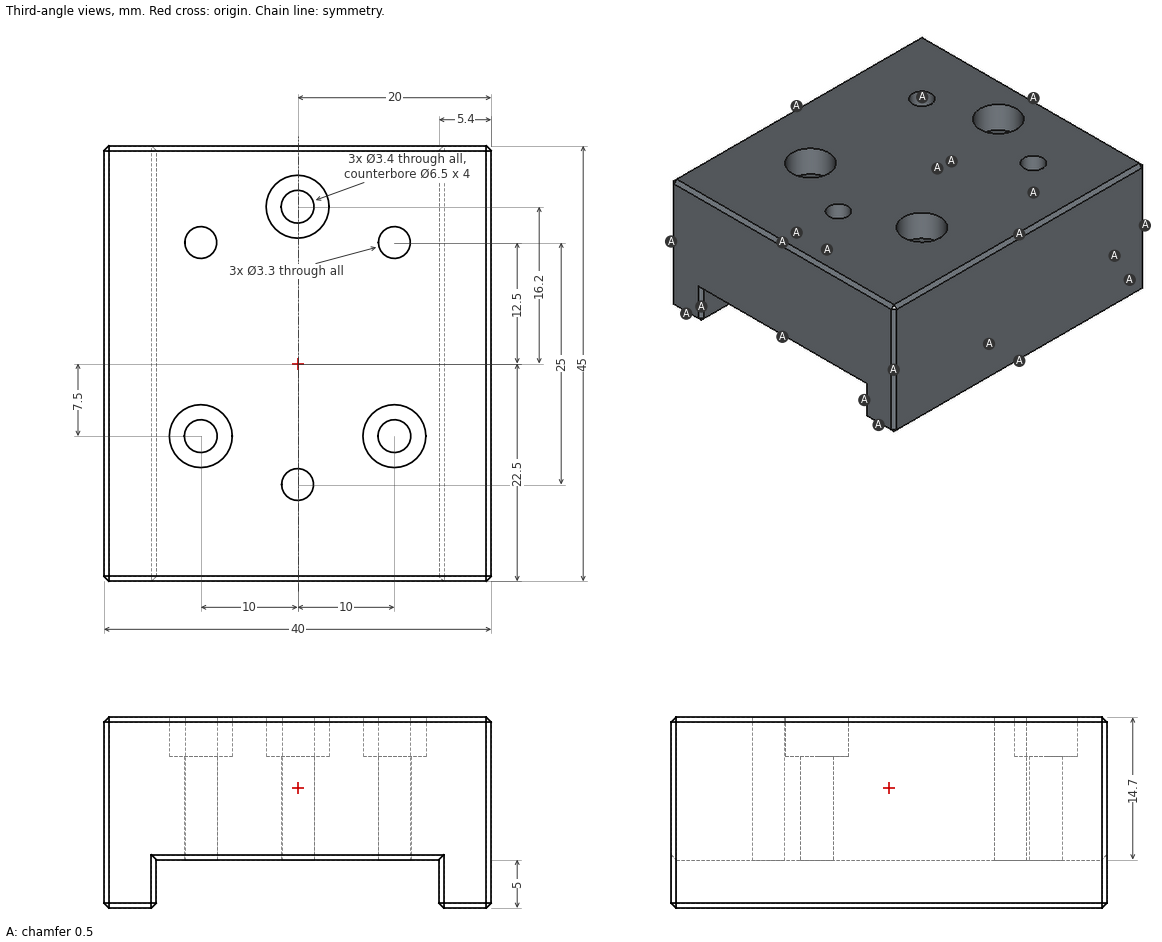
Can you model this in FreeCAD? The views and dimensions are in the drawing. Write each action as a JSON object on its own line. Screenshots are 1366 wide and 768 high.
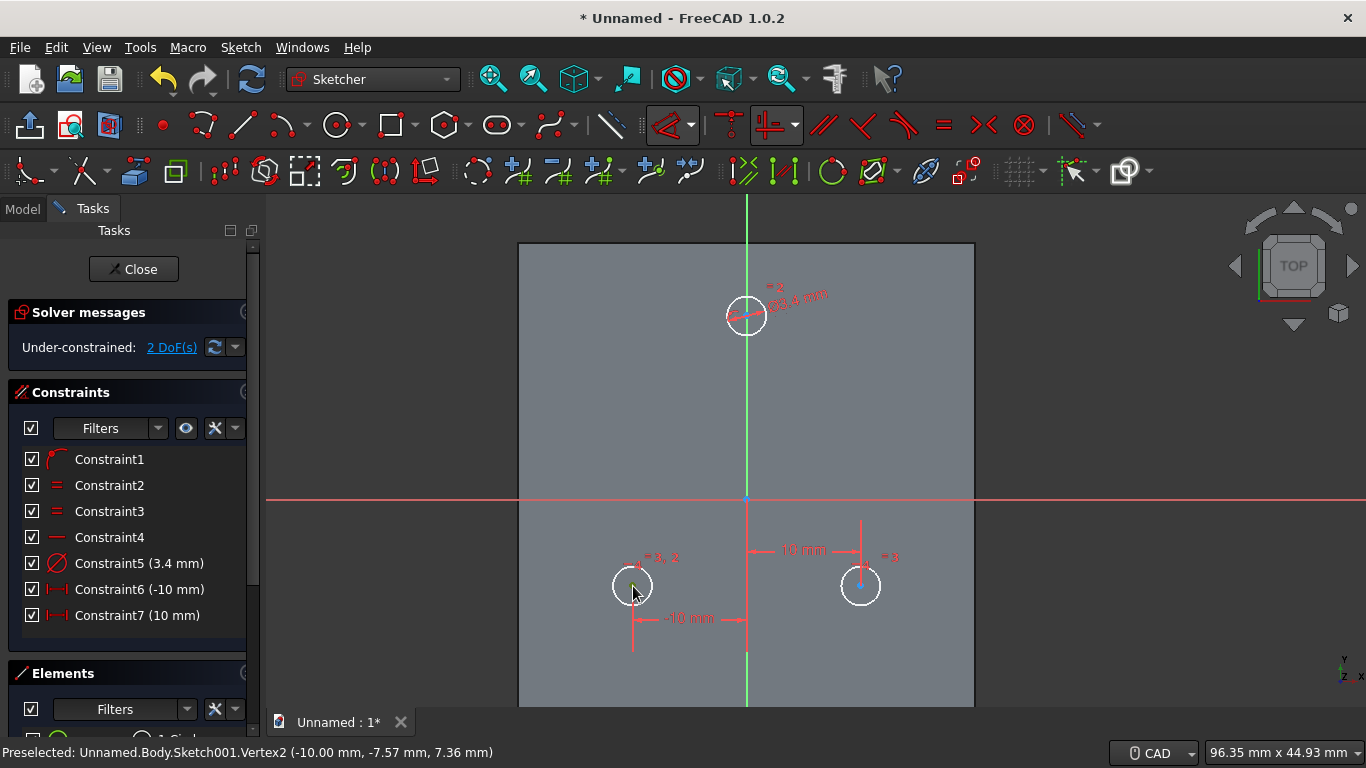
{"action": "key", "text": "i"}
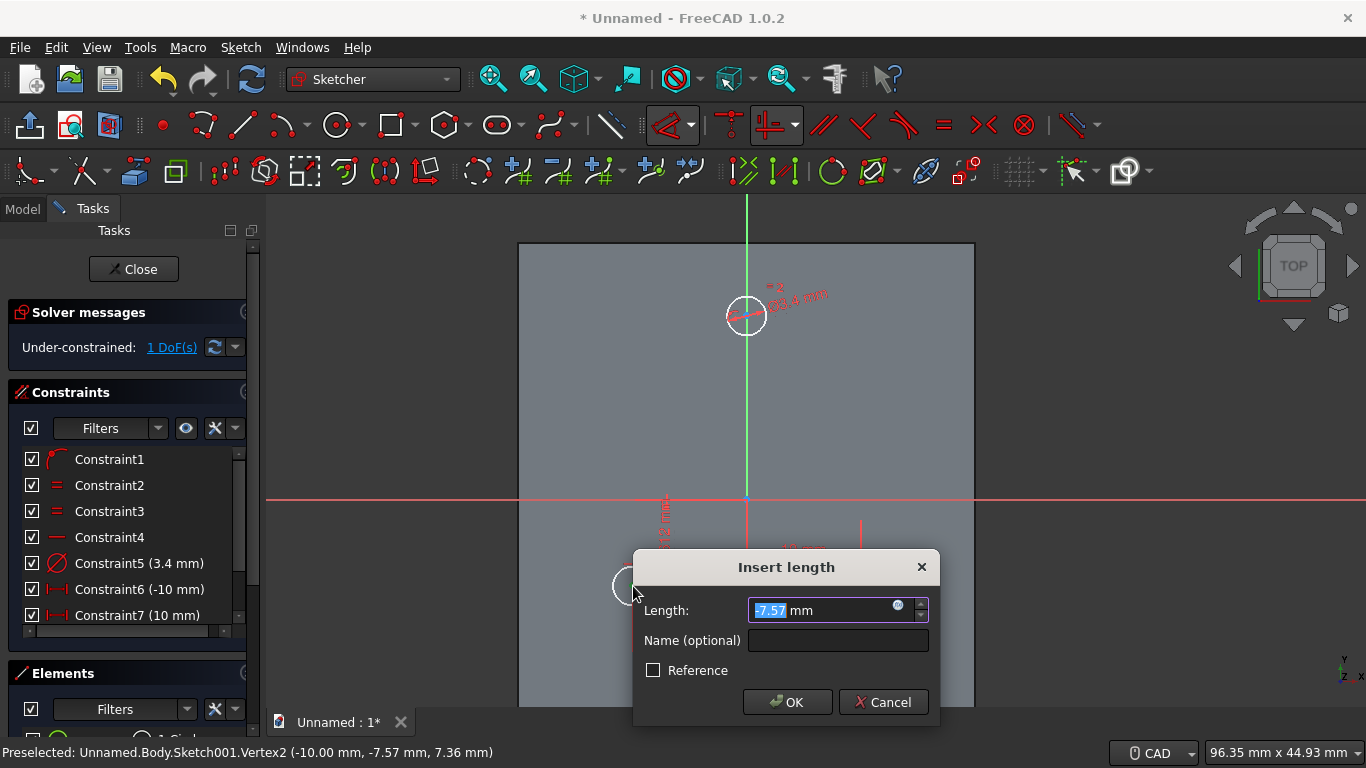
{"action": "type", "text": "-7.5"}
{"action": "key", "text": "Return"}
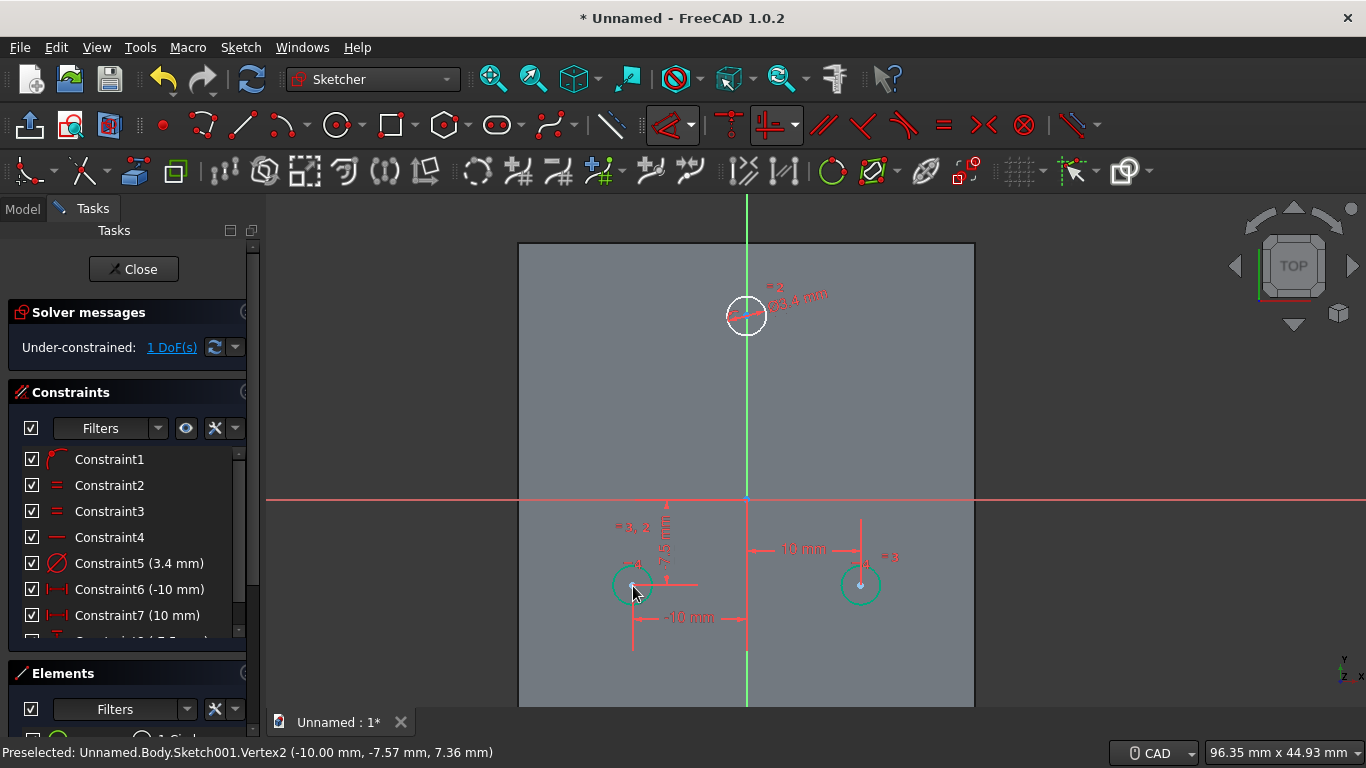
{"action": "left_click", "coordinate": [747, 316]}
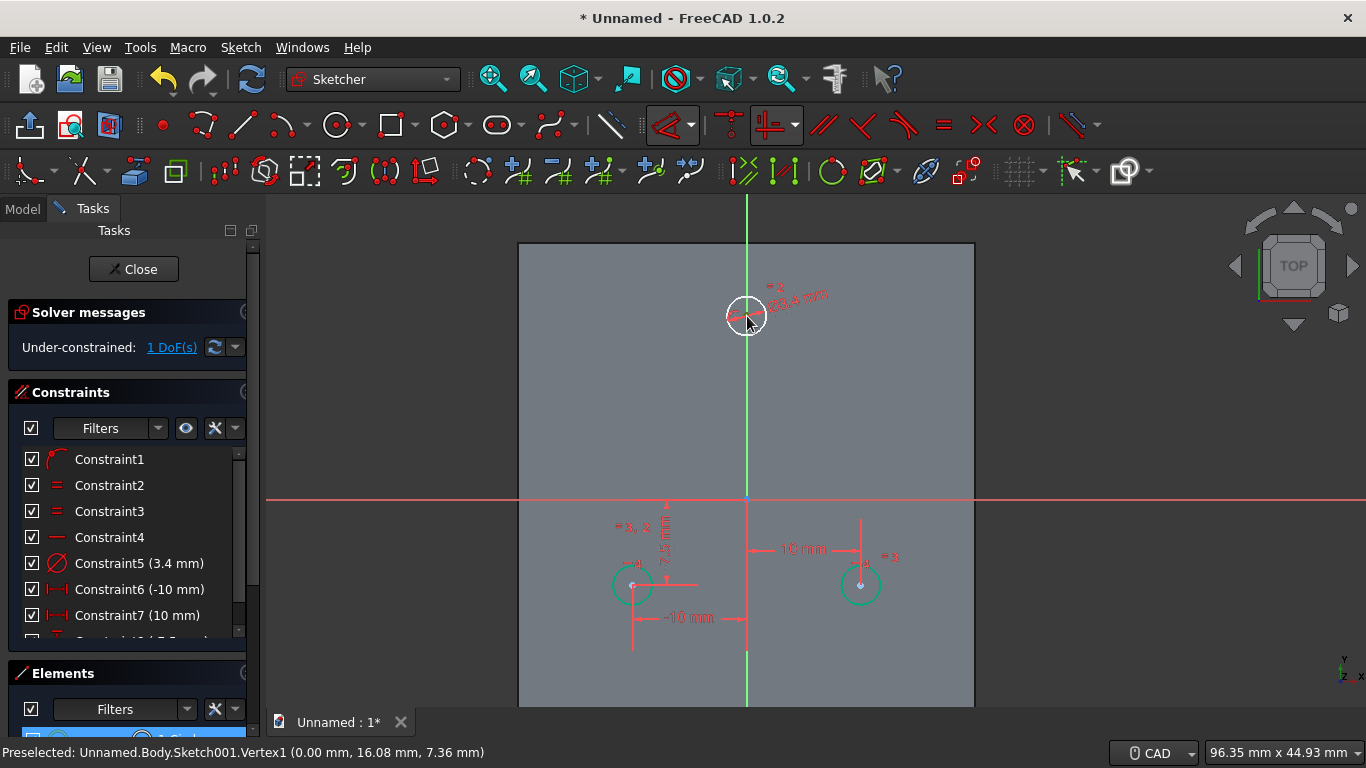
{"action": "left_click", "coordinate": [694, 126]}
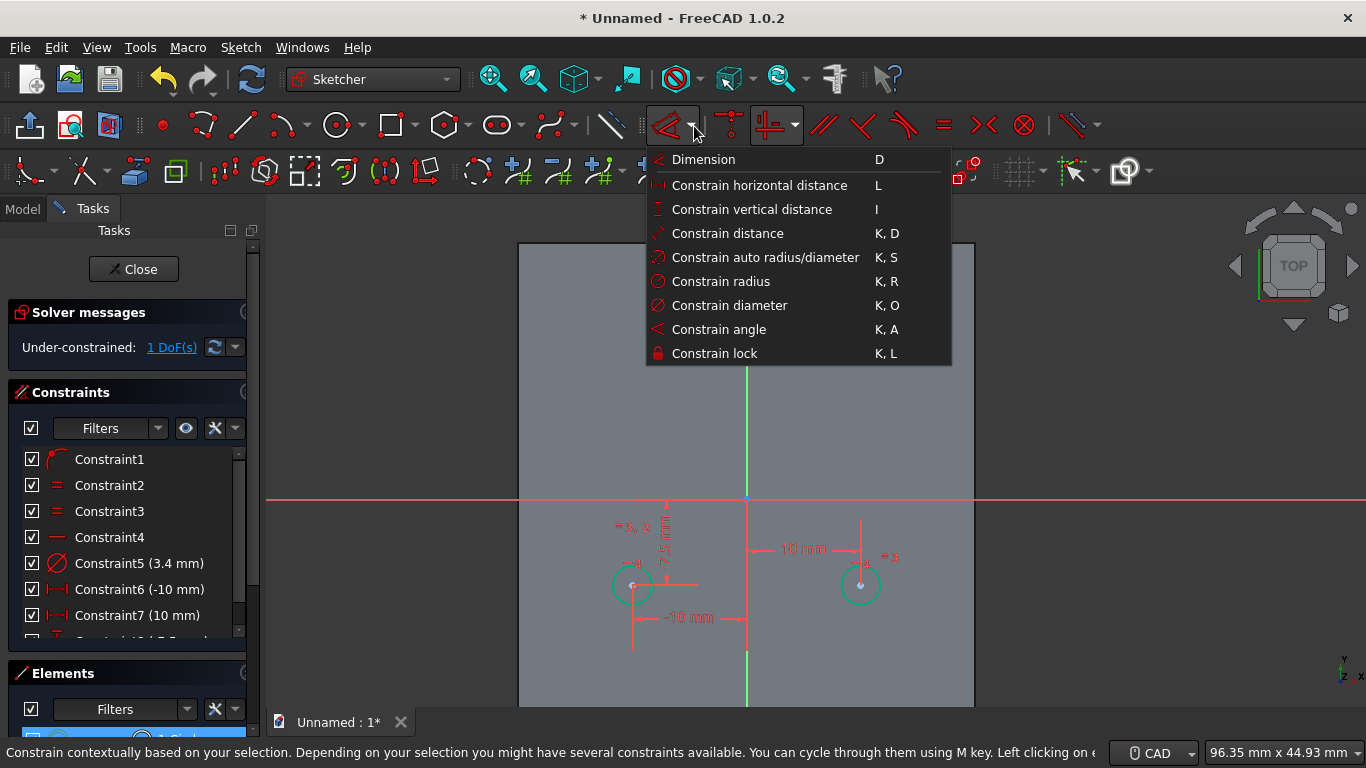
{"action": "left_click", "coordinate": [799, 209]}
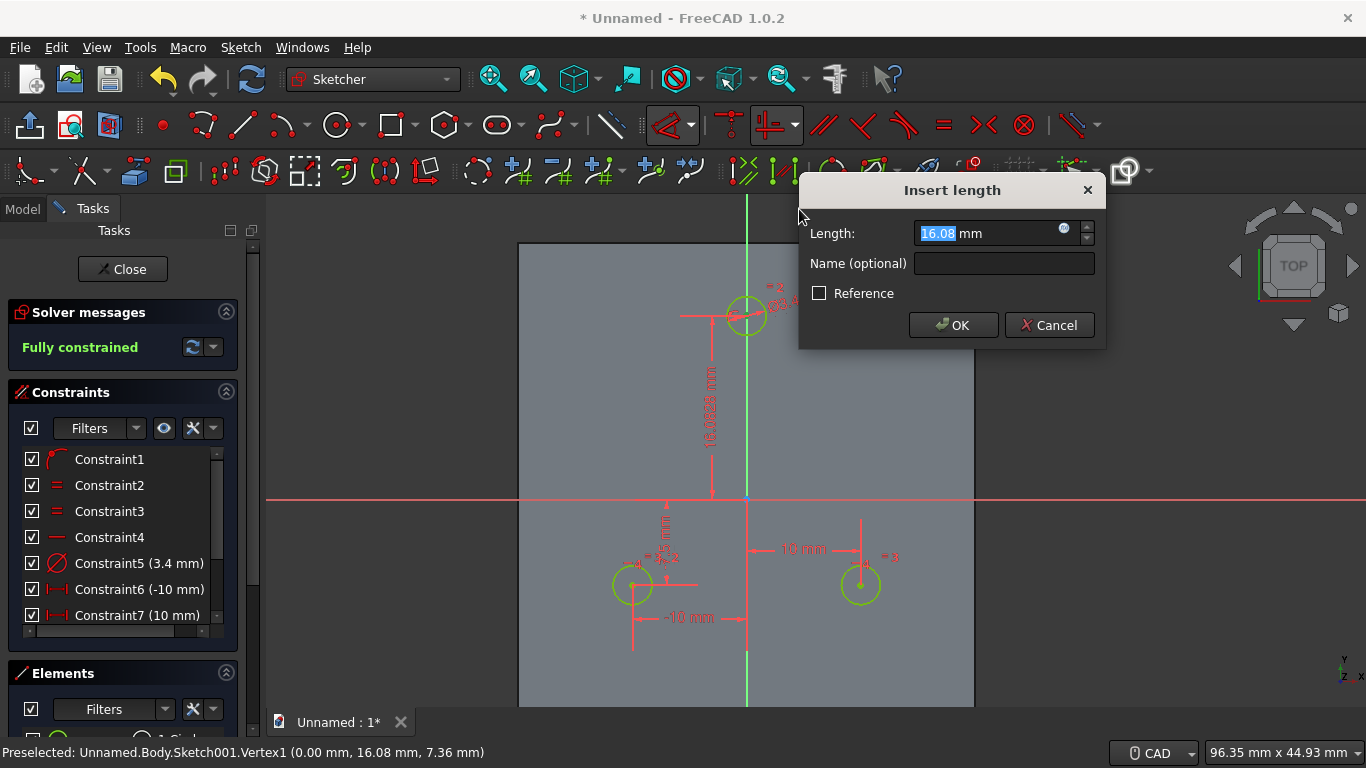
{"action": "type", "text": "16.2"}
{"action": "key", "text": "Return"}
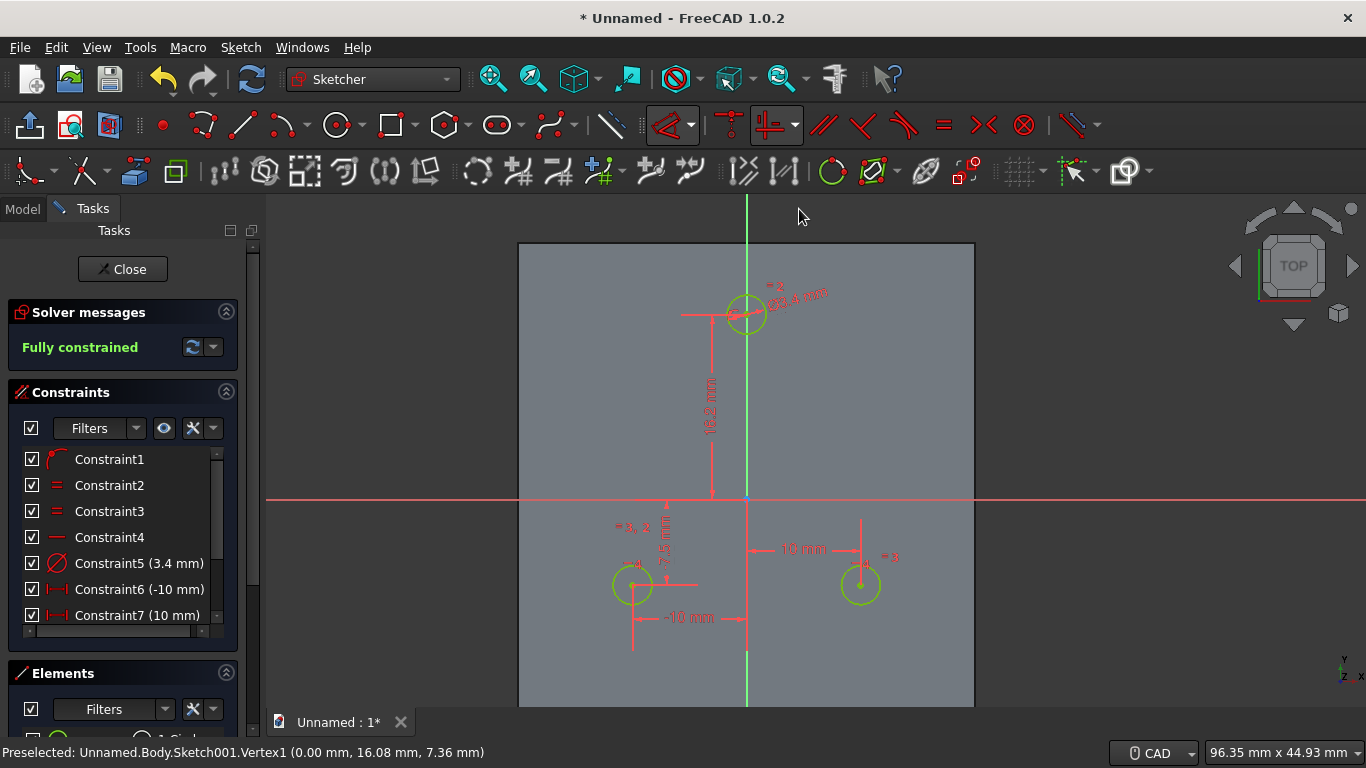
{"action": "left_click", "coordinate": [123, 269]}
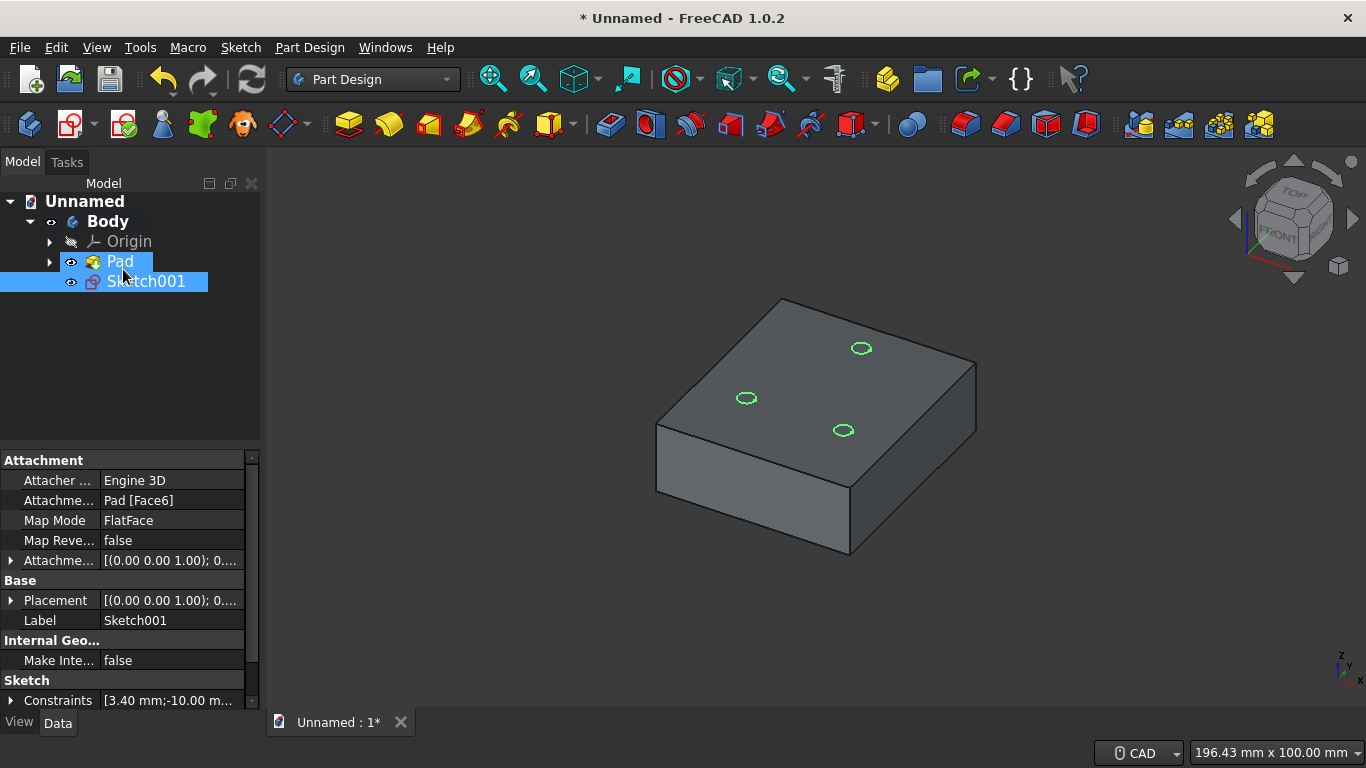
{"action": "left_click", "coordinate": [652, 124]}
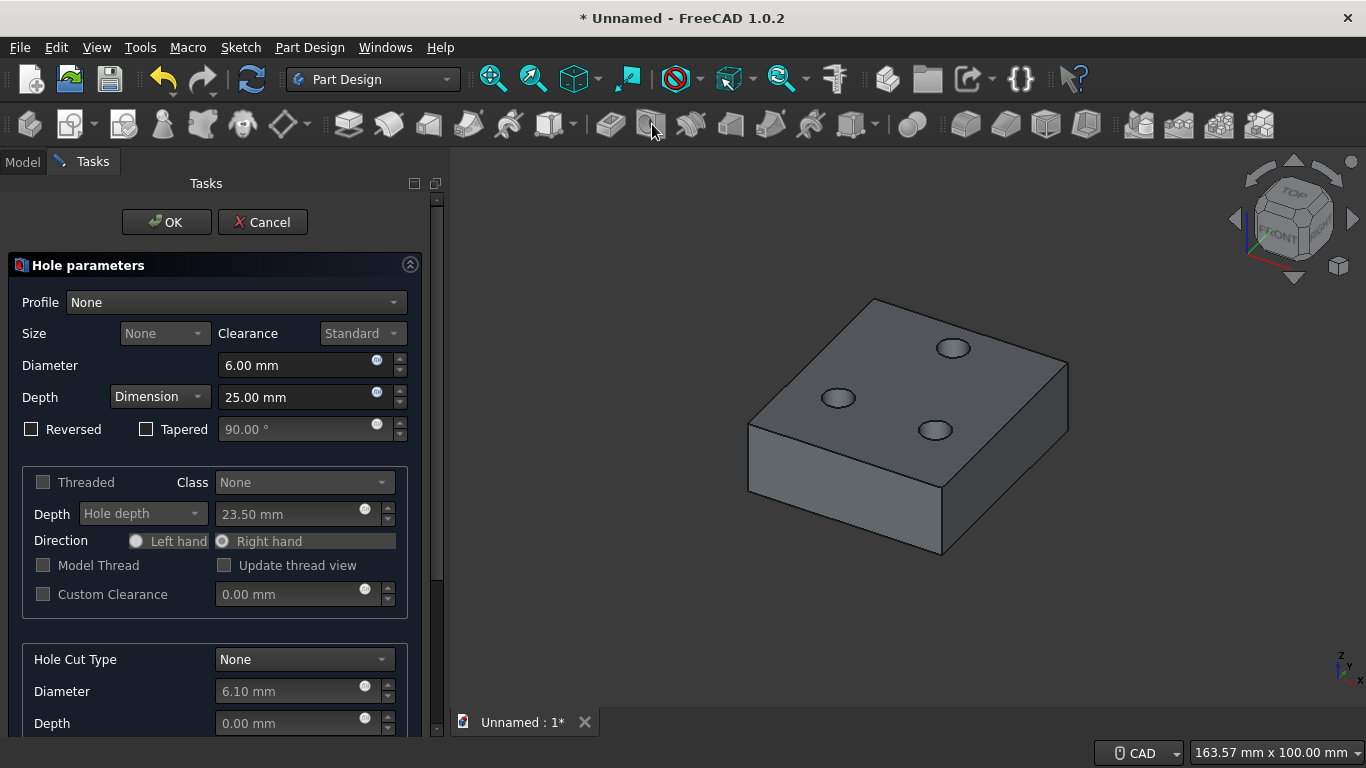
{"action": "triple_click", "coordinate": [305, 365]}